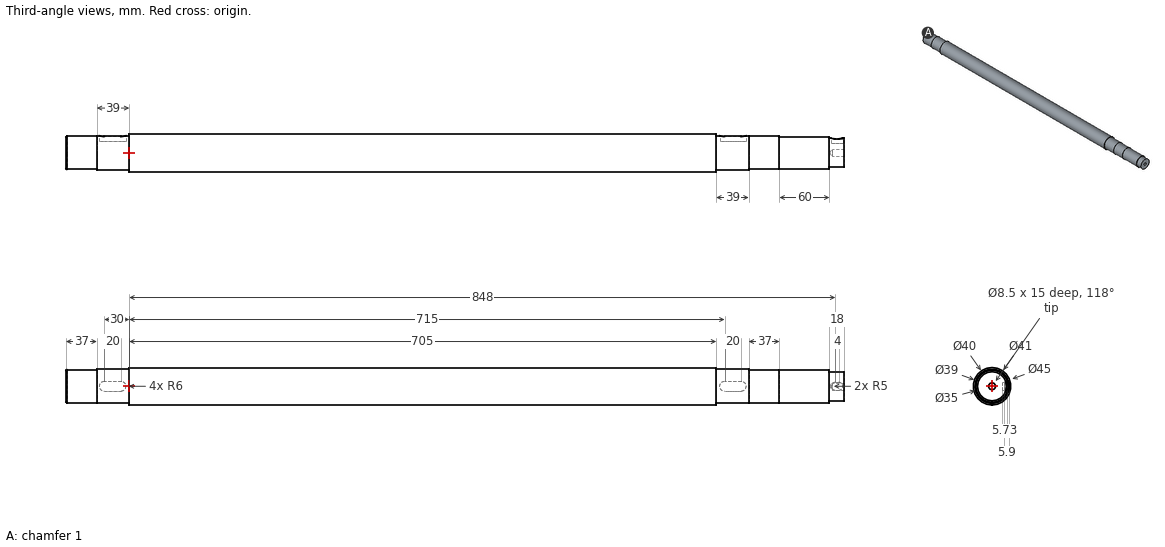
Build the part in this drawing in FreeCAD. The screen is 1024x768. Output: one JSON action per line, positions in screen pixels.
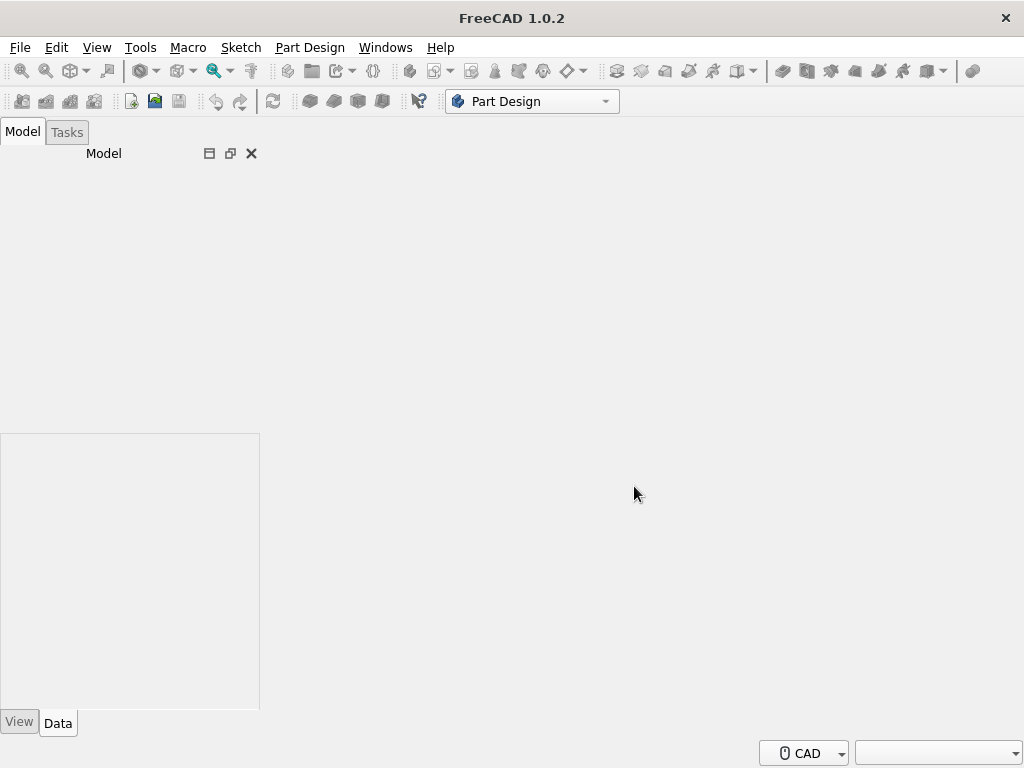
{"action": "left_click", "coordinate": [132, 102]}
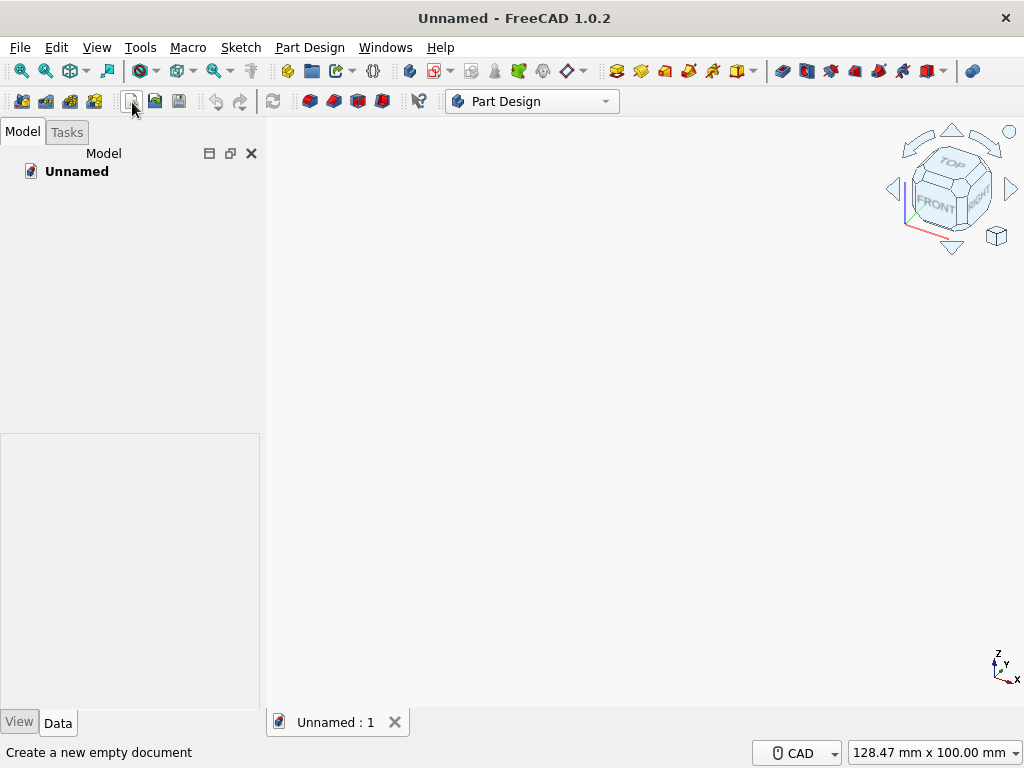
{"action": "left_click", "coordinate": [434, 72]}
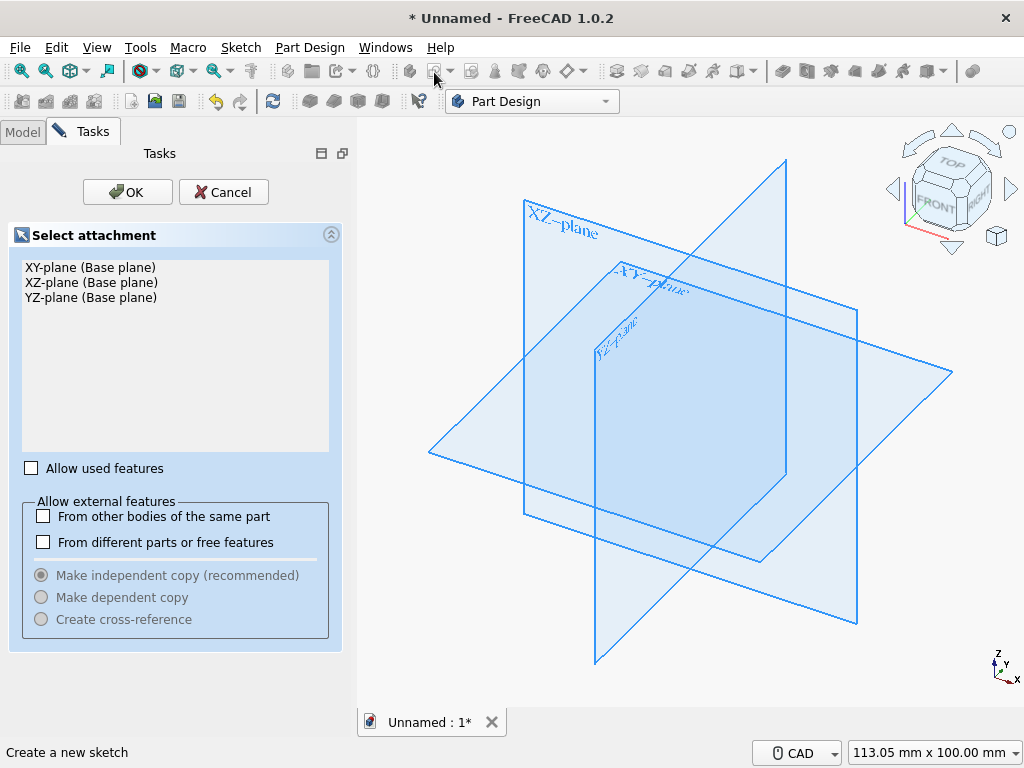
{"action": "left_click", "coordinate": [82, 298]}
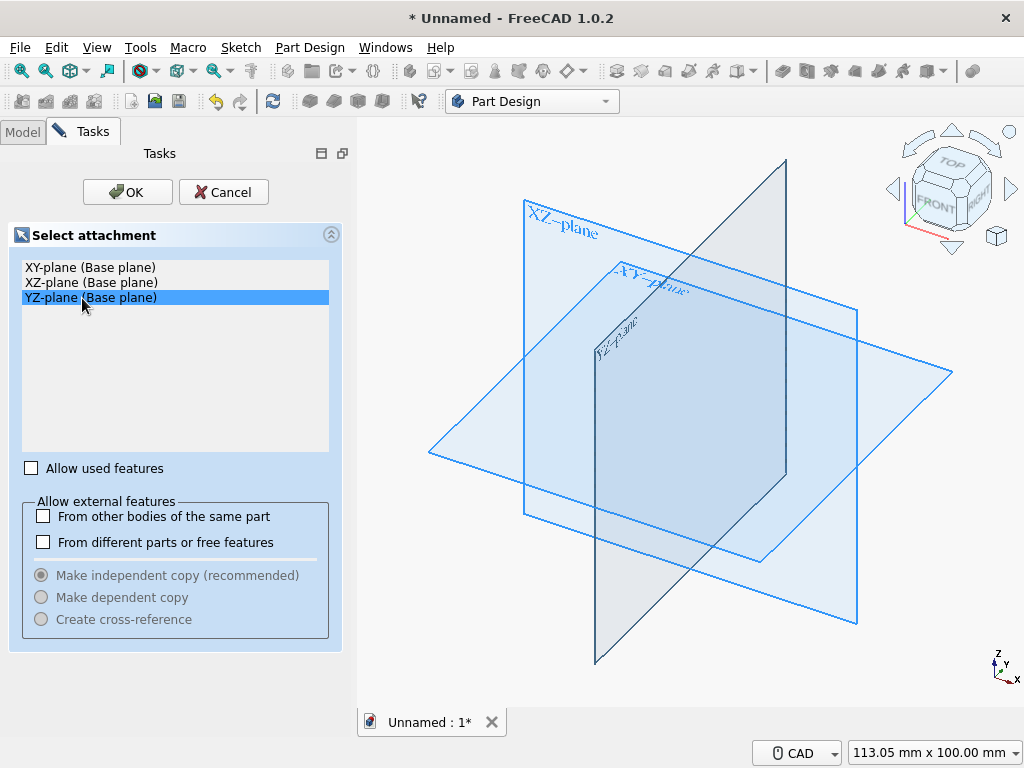
{"action": "left_click", "coordinate": [128, 192]}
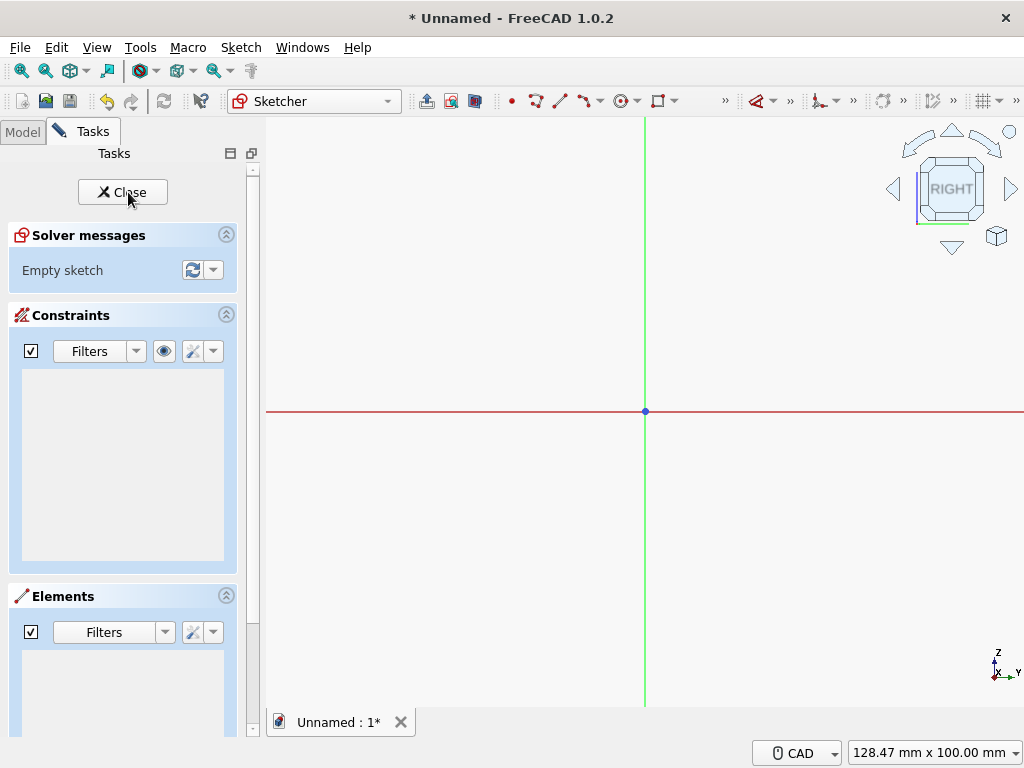
{"action": "scroll", "coordinate": [784, 412], "scroll_direction": "up", "scroll_amount": 2}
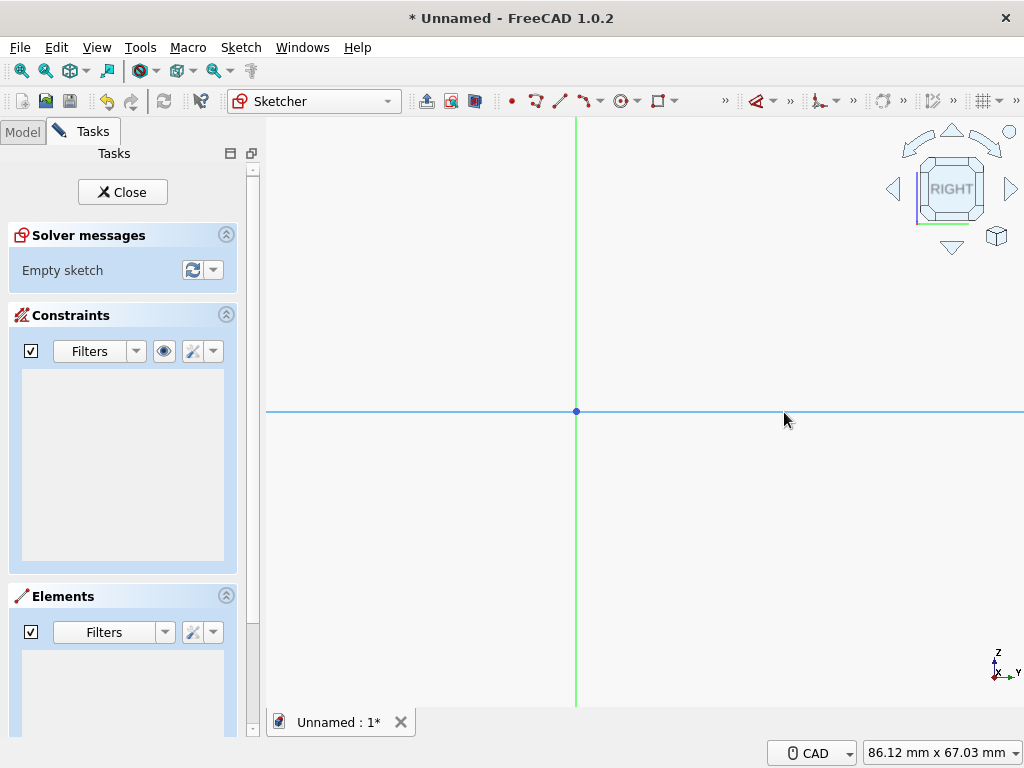
{"action": "left_click", "coordinate": [622, 102]}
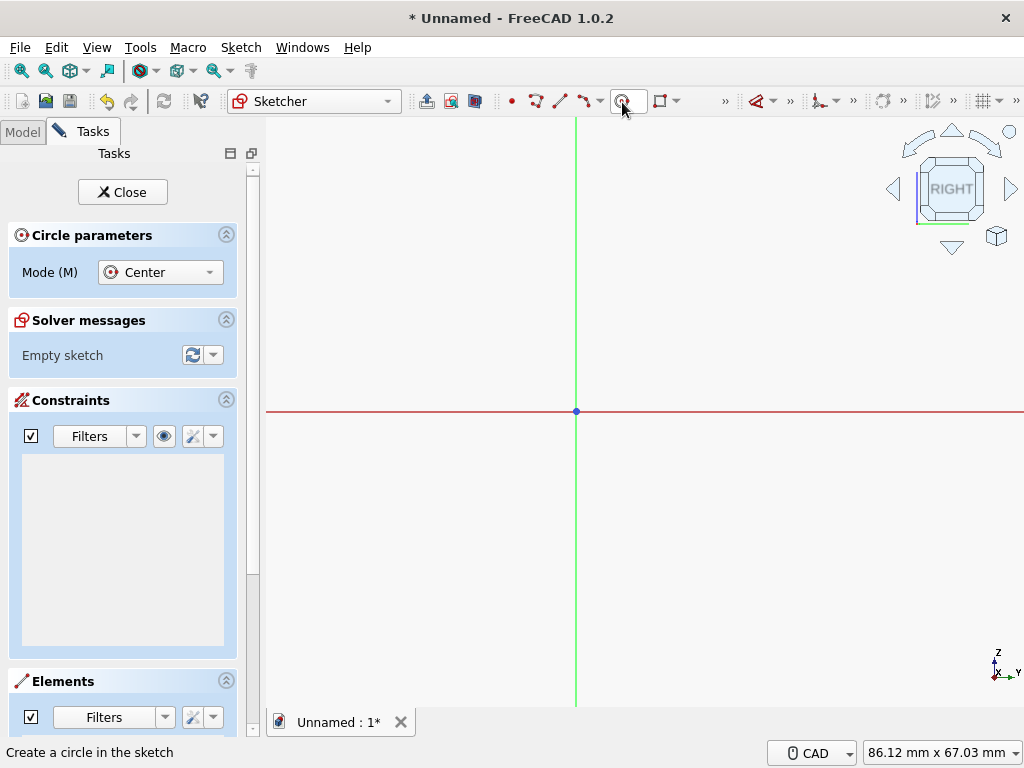
{"action": "left_click", "coordinate": [576, 412]}
{"action": "mouse_move", "coordinate": [716, 272]}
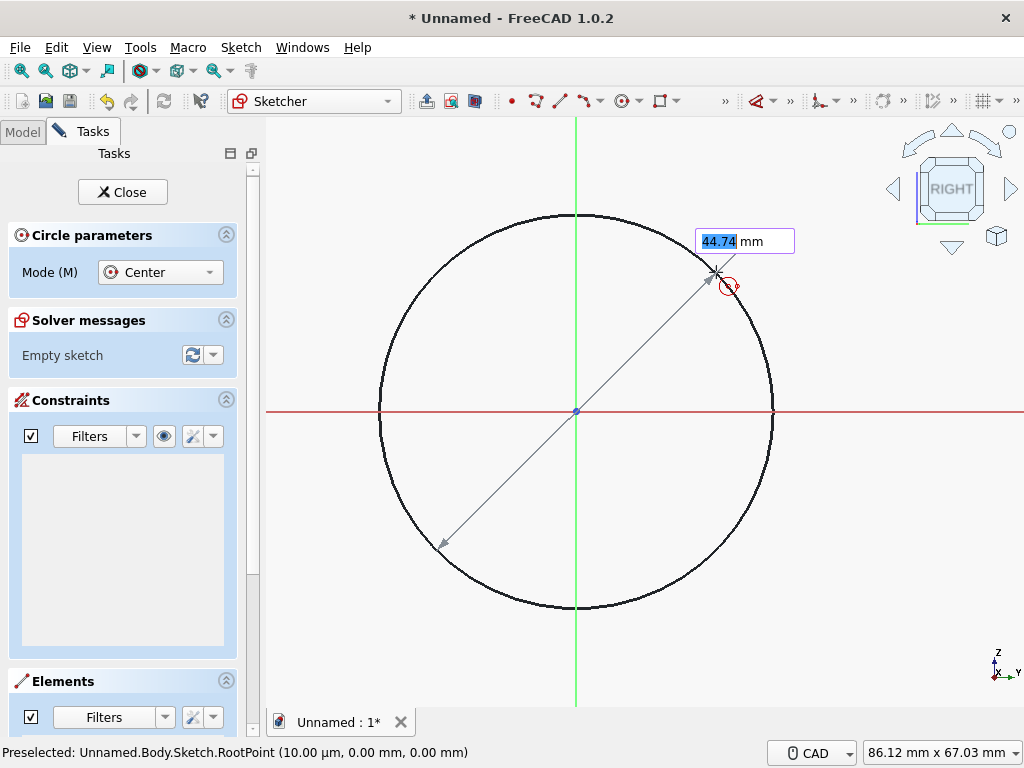
{"action": "type", "text": "45"}
{"action": "key", "text": "Return"}
{"action": "key", "text": "Escape"}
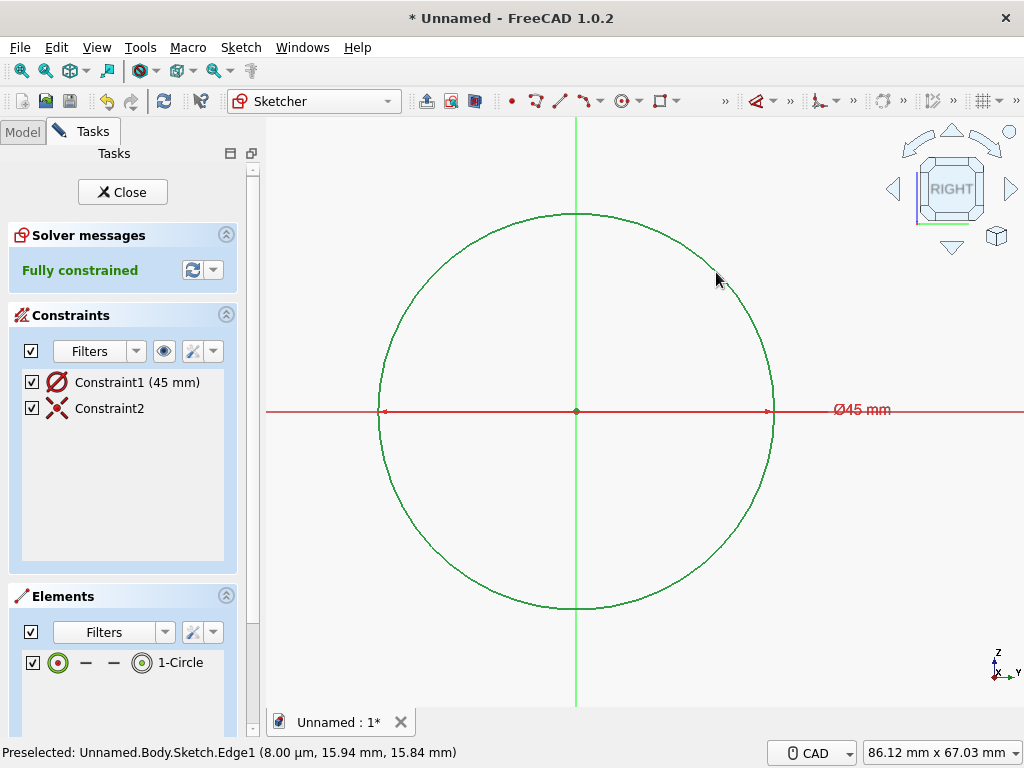
{"action": "left_click", "coordinate": [123, 192]}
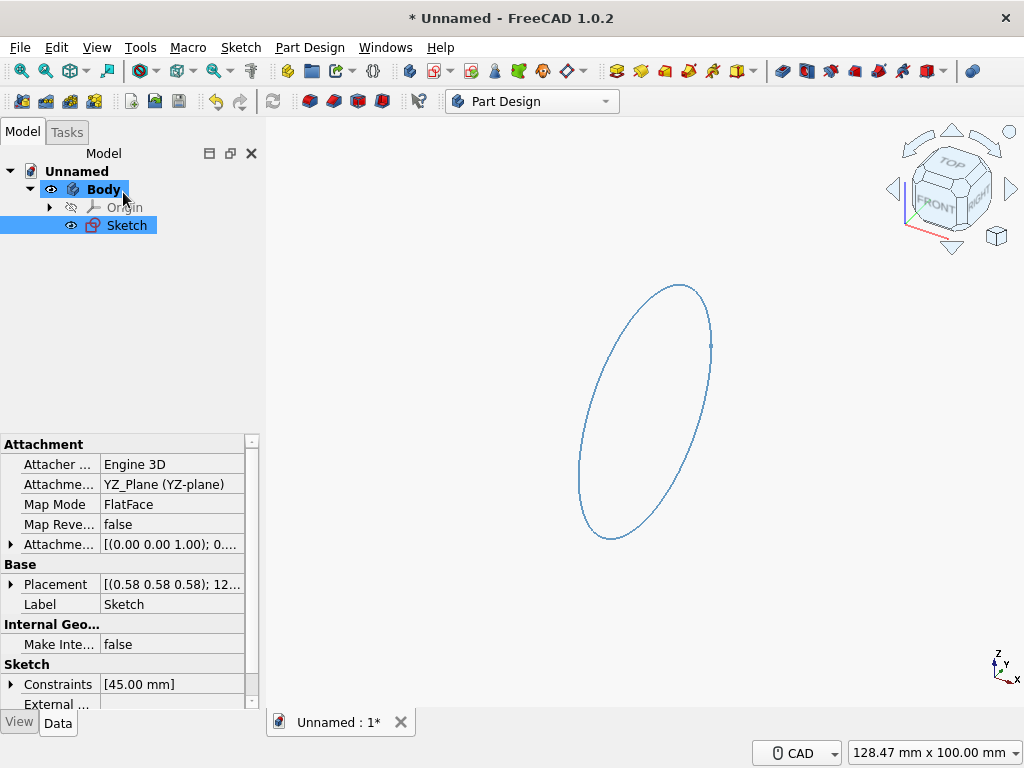
{"action": "left_click", "coordinate": [618, 72]}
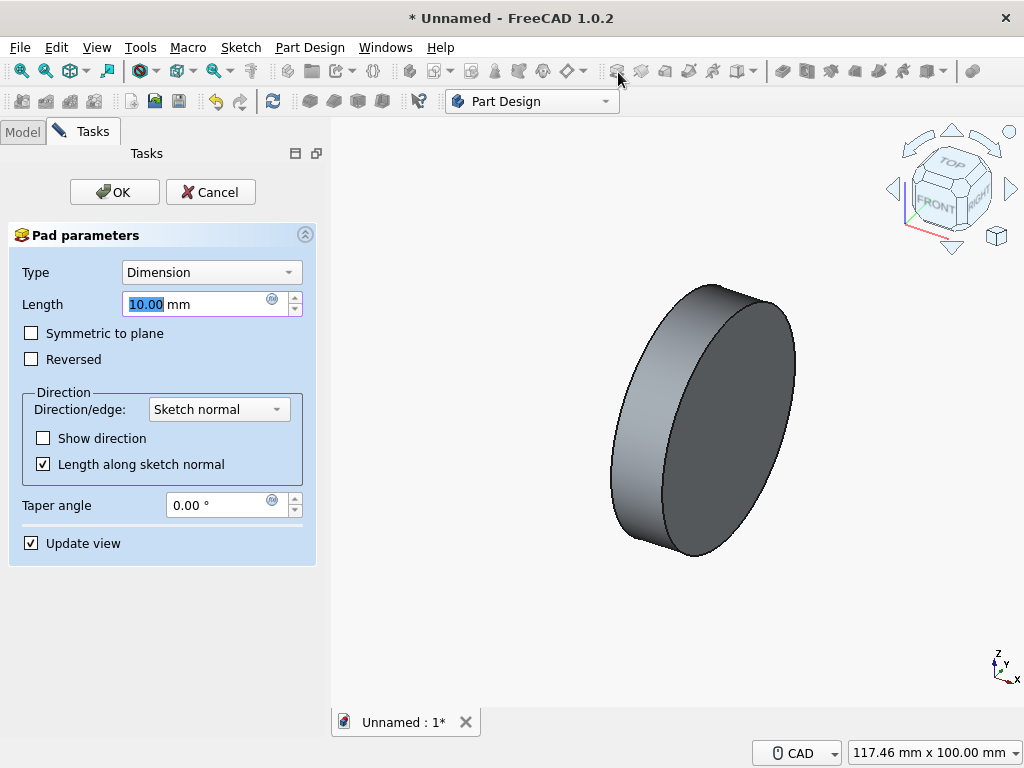
{"action": "type", "text": "705"}
{"action": "key", "text": "Tab"}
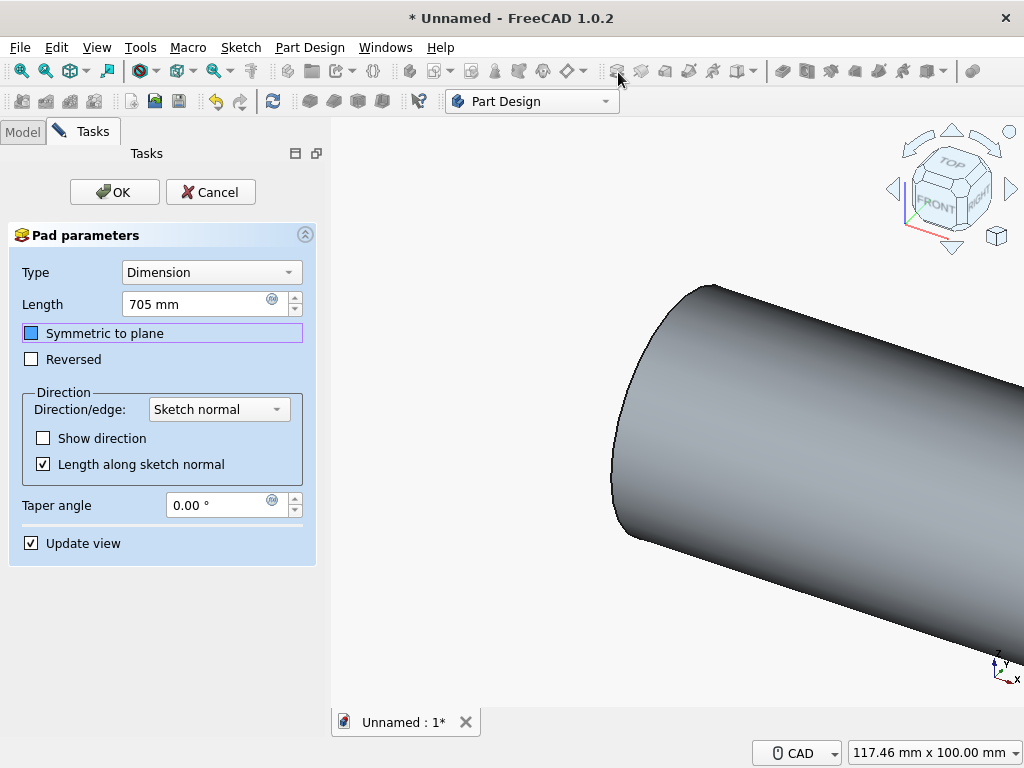
{"action": "left_click", "coordinate": [115, 192]}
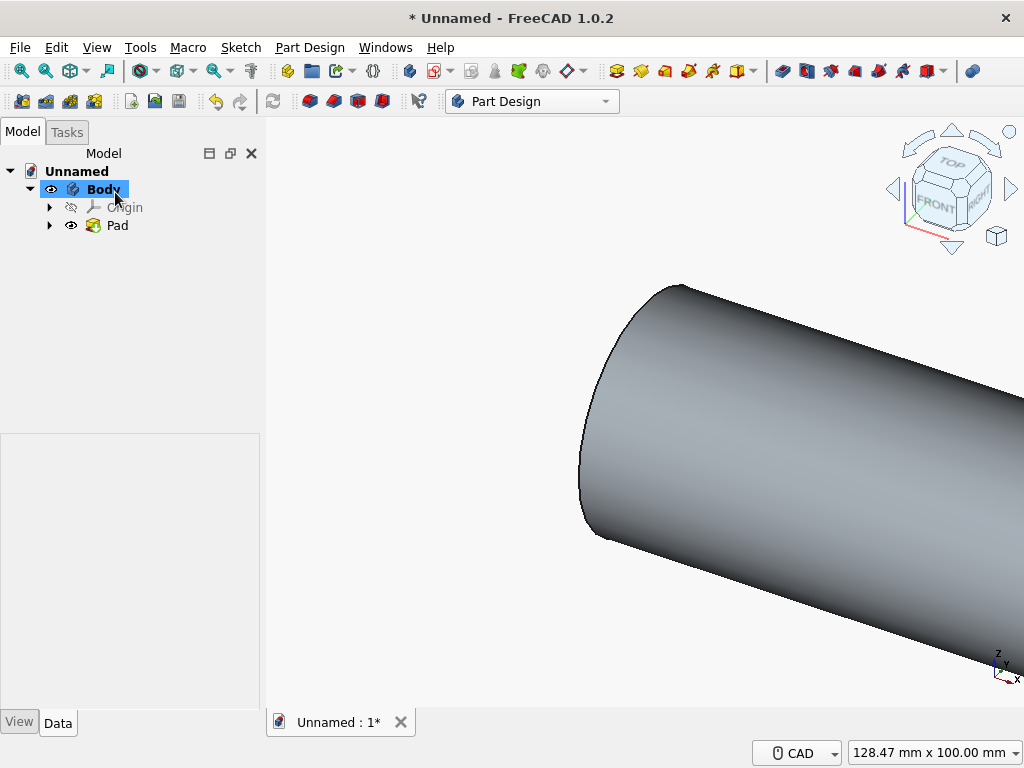
{"action": "left_click", "coordinate": [22, 72]}